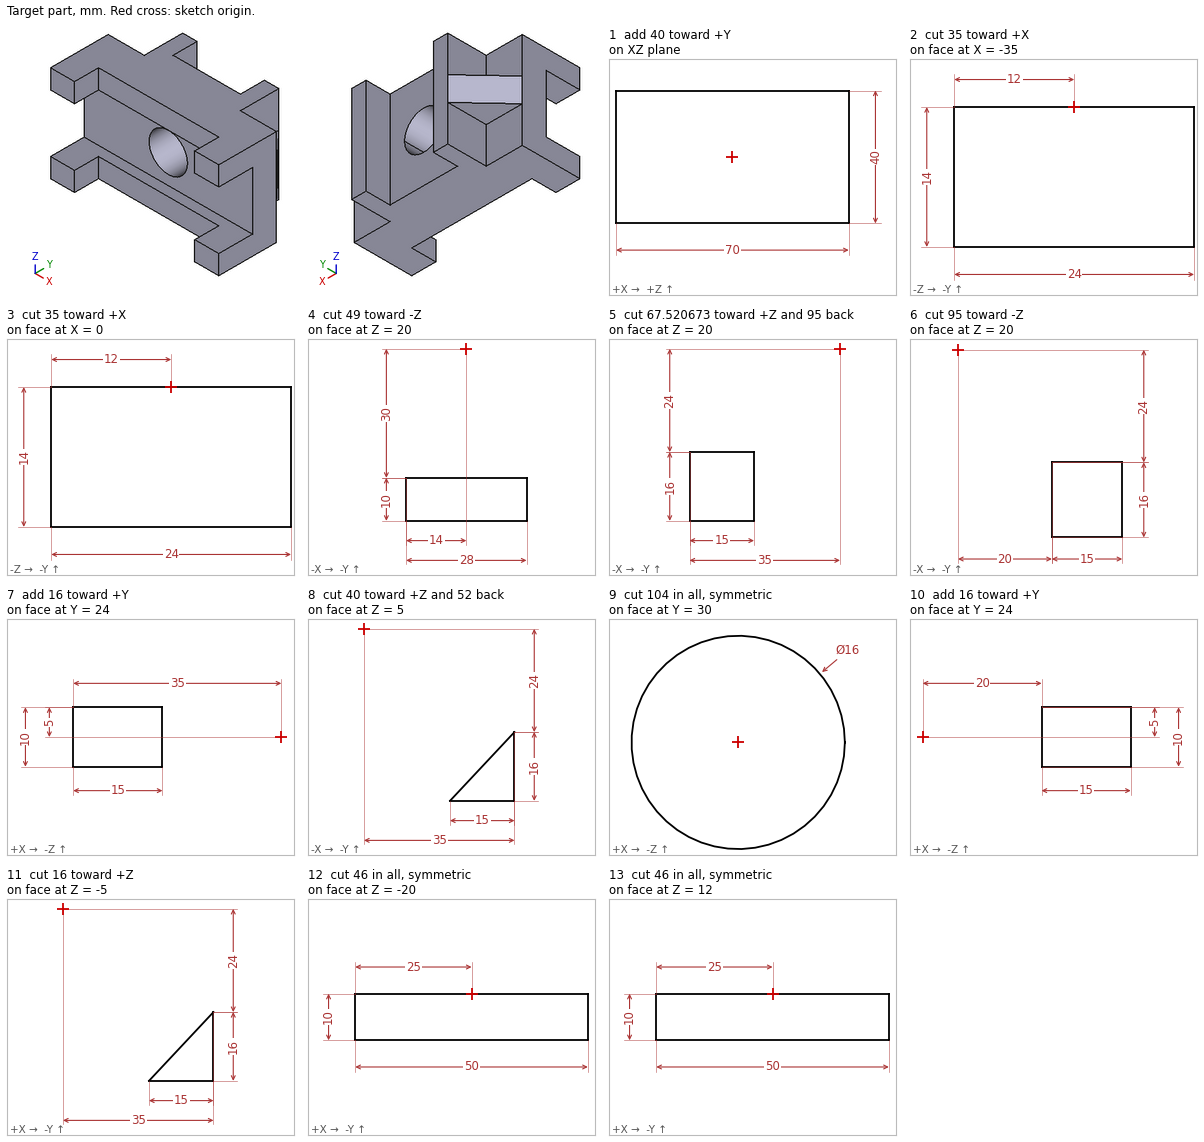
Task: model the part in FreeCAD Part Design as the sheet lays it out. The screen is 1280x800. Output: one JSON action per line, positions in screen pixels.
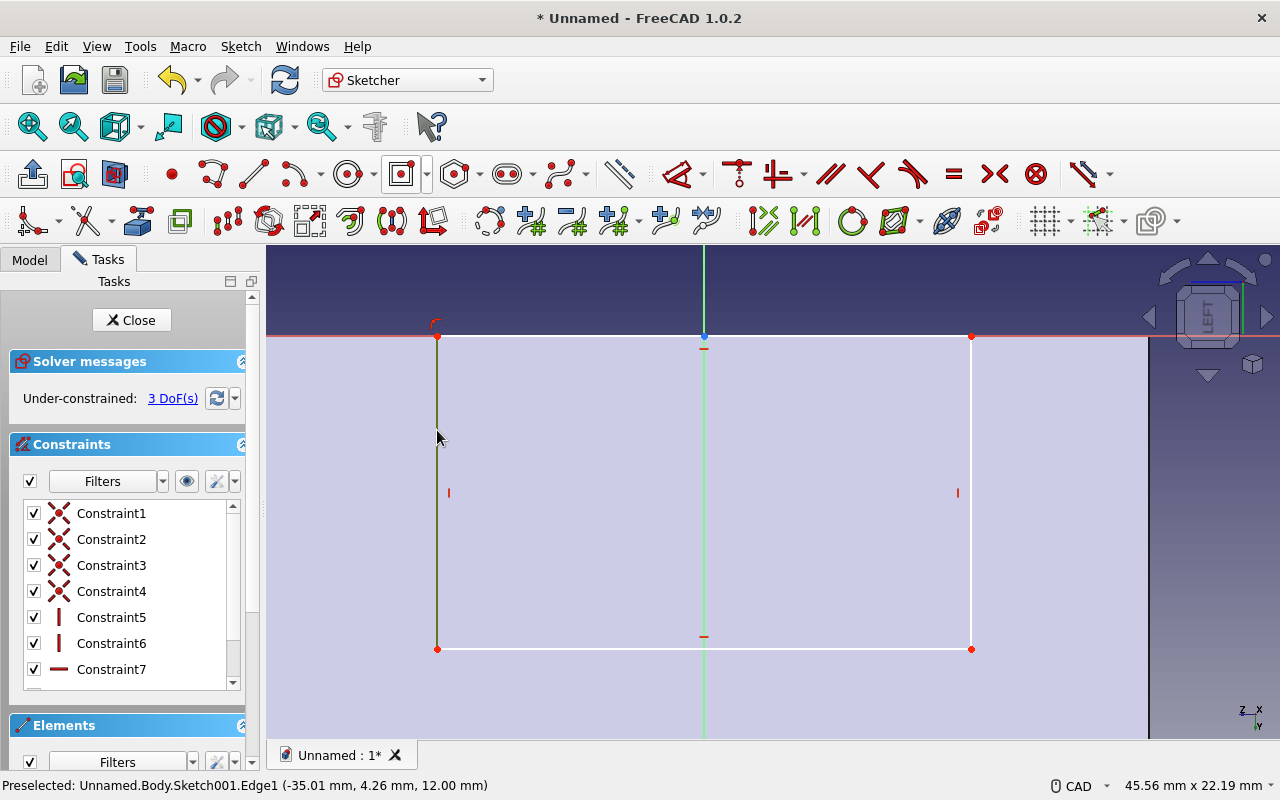
{"action": "key", "text": "i"}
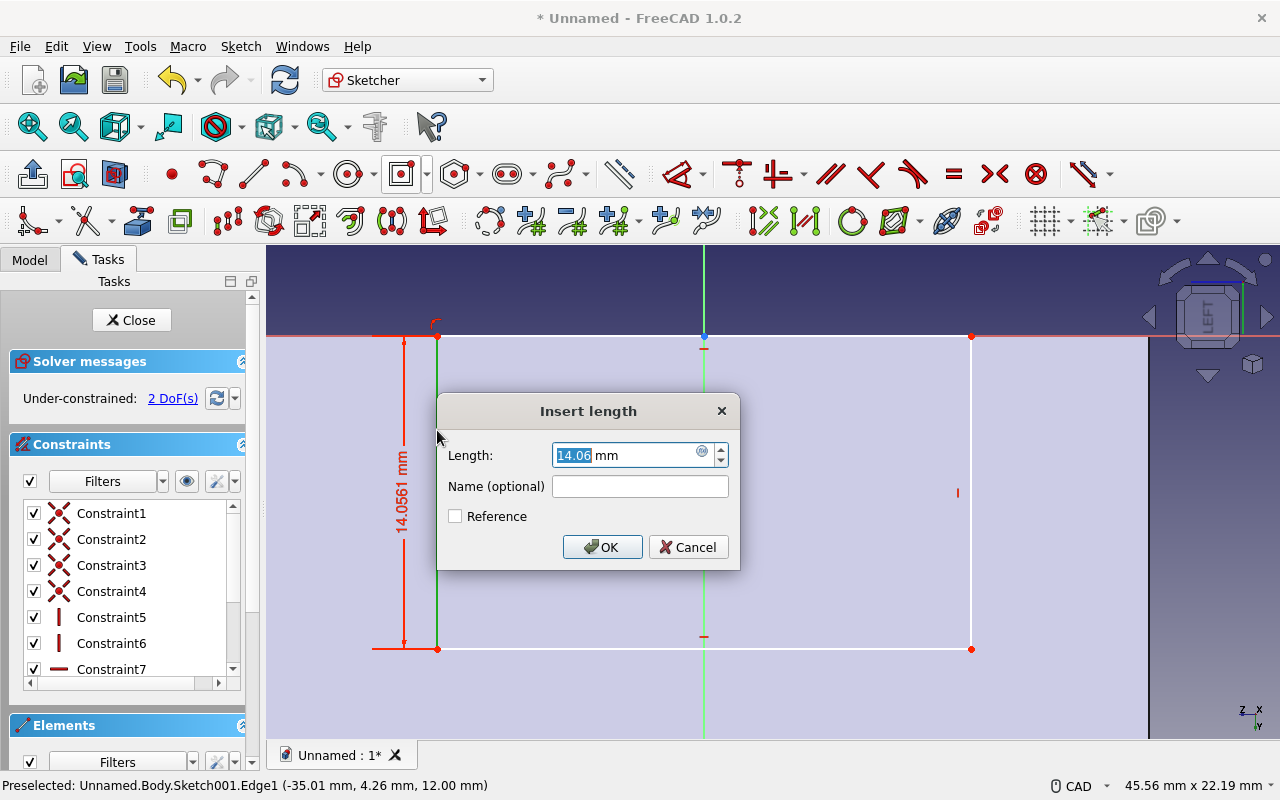
{"action": "type", "text": "14"}
{"action": "key", "text": "Return"}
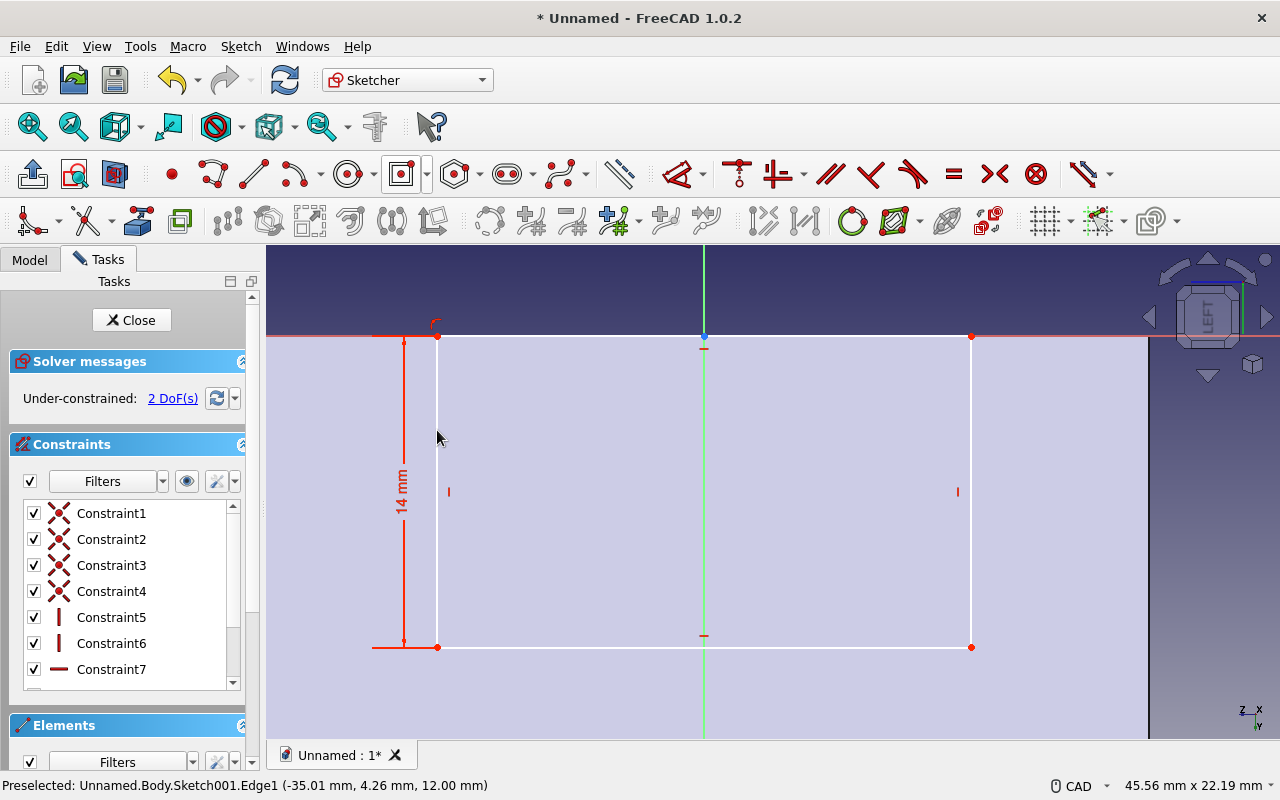
{"action": "left_click", "coordinate": [597, 648]}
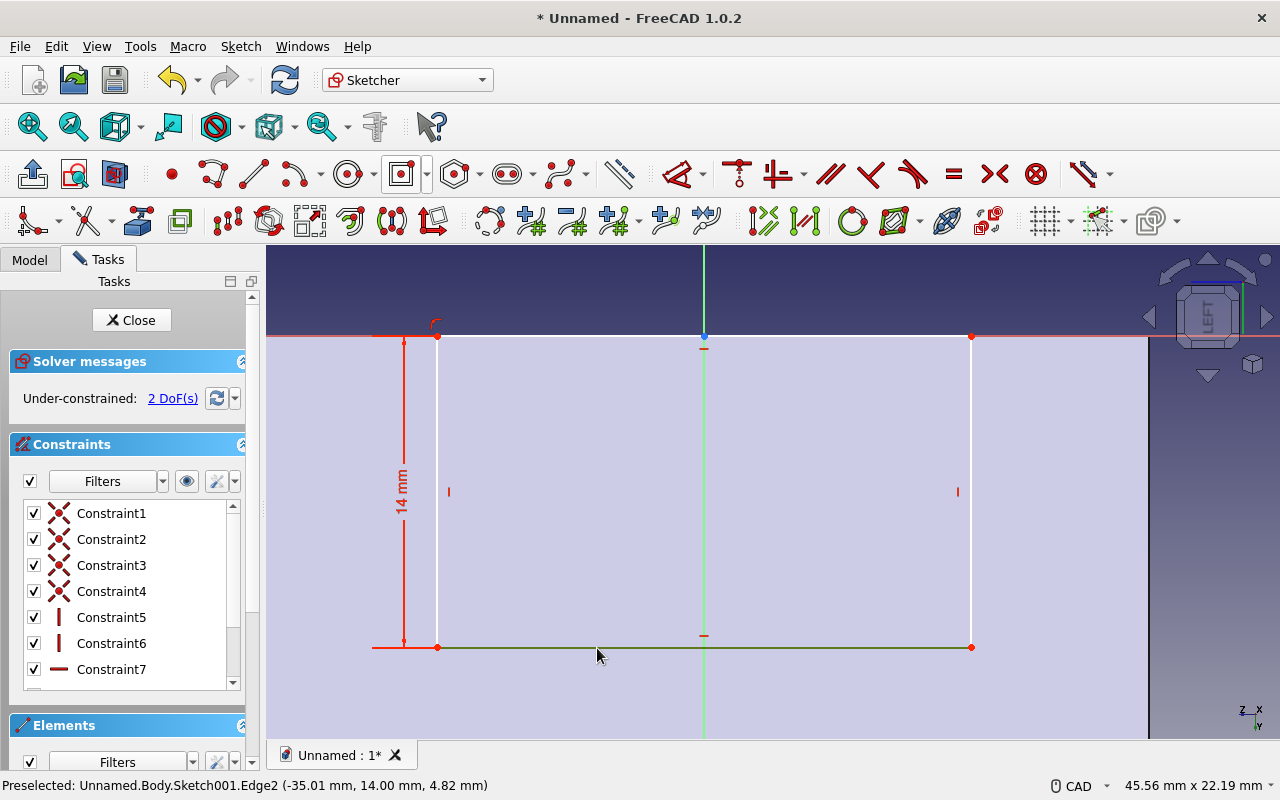
{"action": "key", "text": "l"}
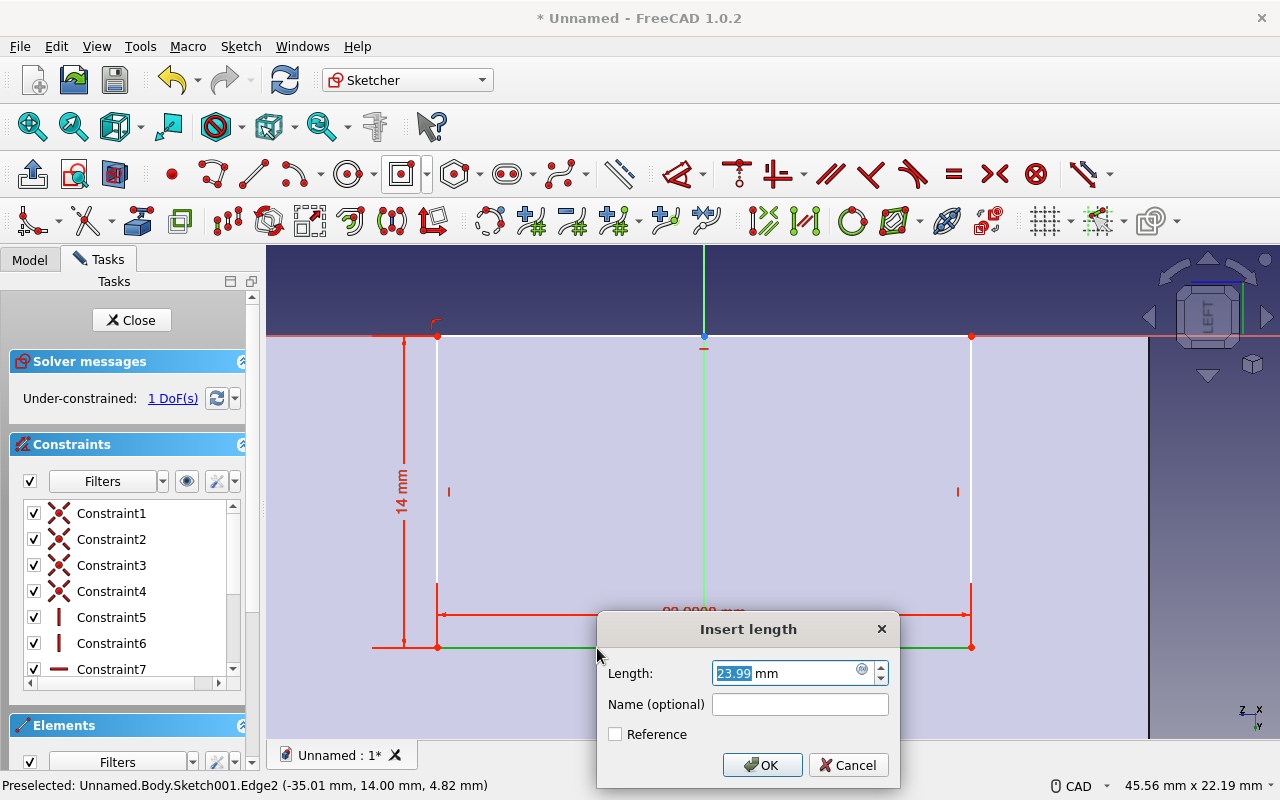
{"action": "type", "text": "24"}
{"action": "key", "text": "Return"}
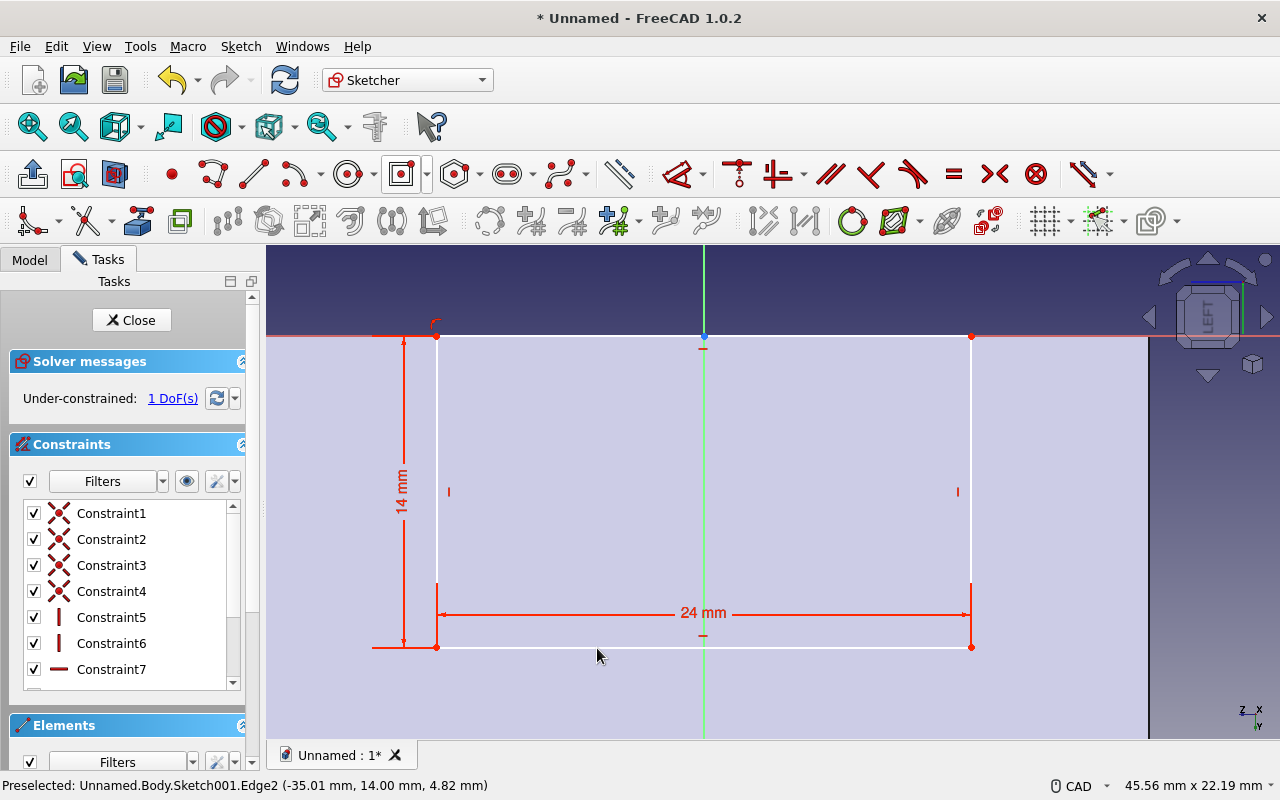
{"action": "left_click", "coordinate": [437, 336]}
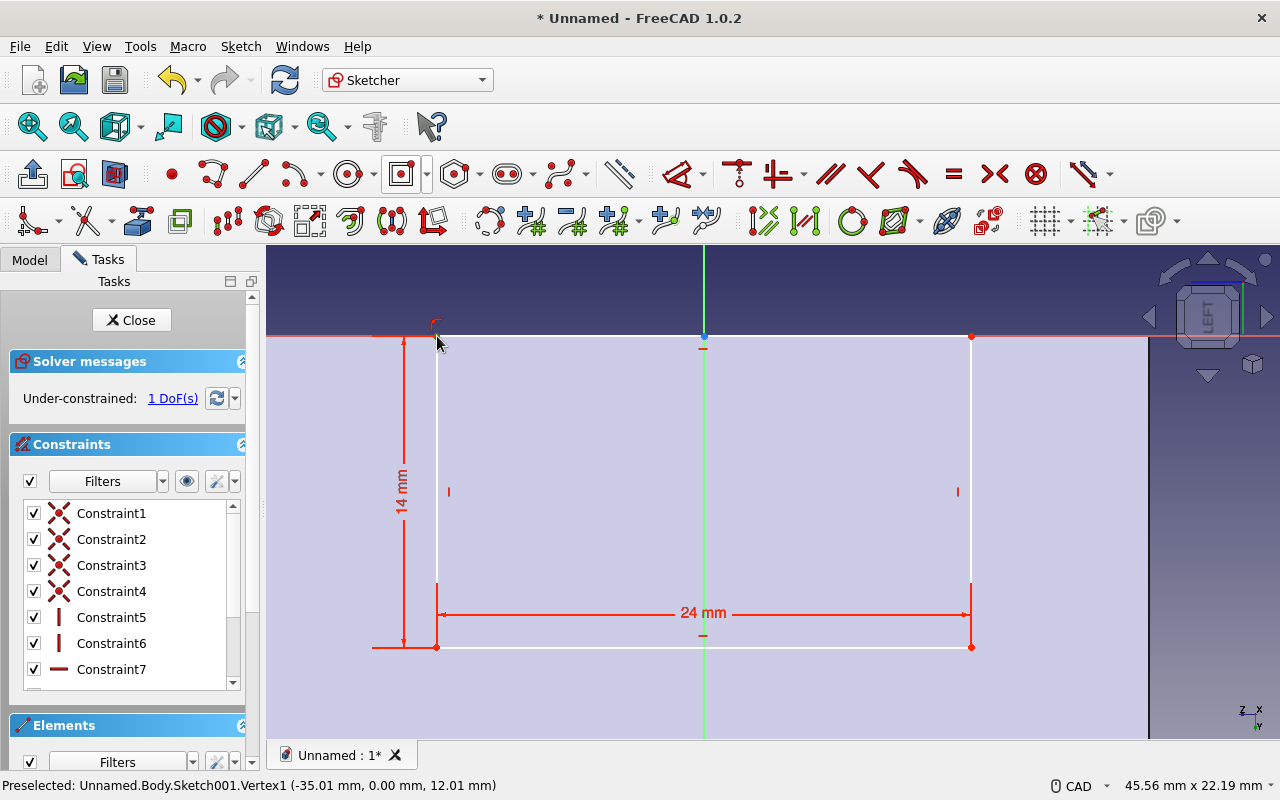
{"action": "key", "text": "l"}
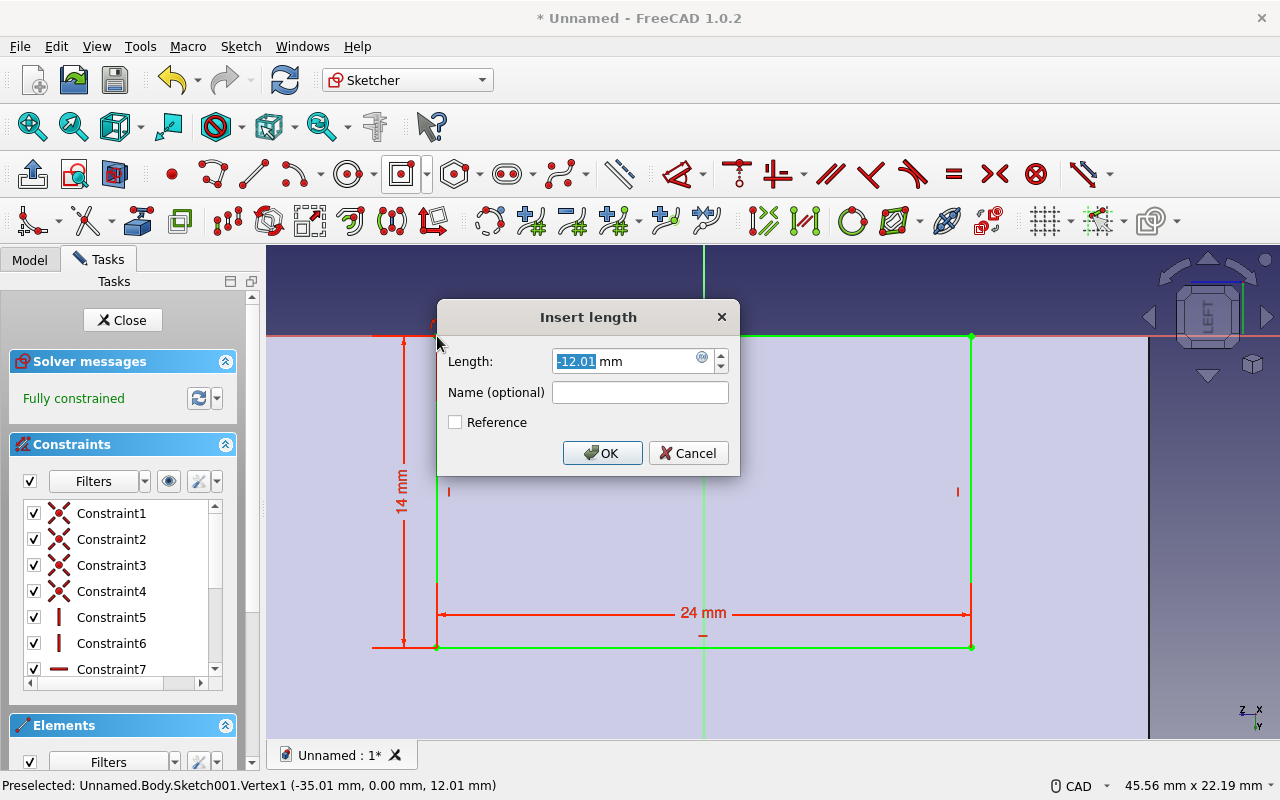
{"action": "type", "text": "-12"}
{"action": "key", "text": "Return"}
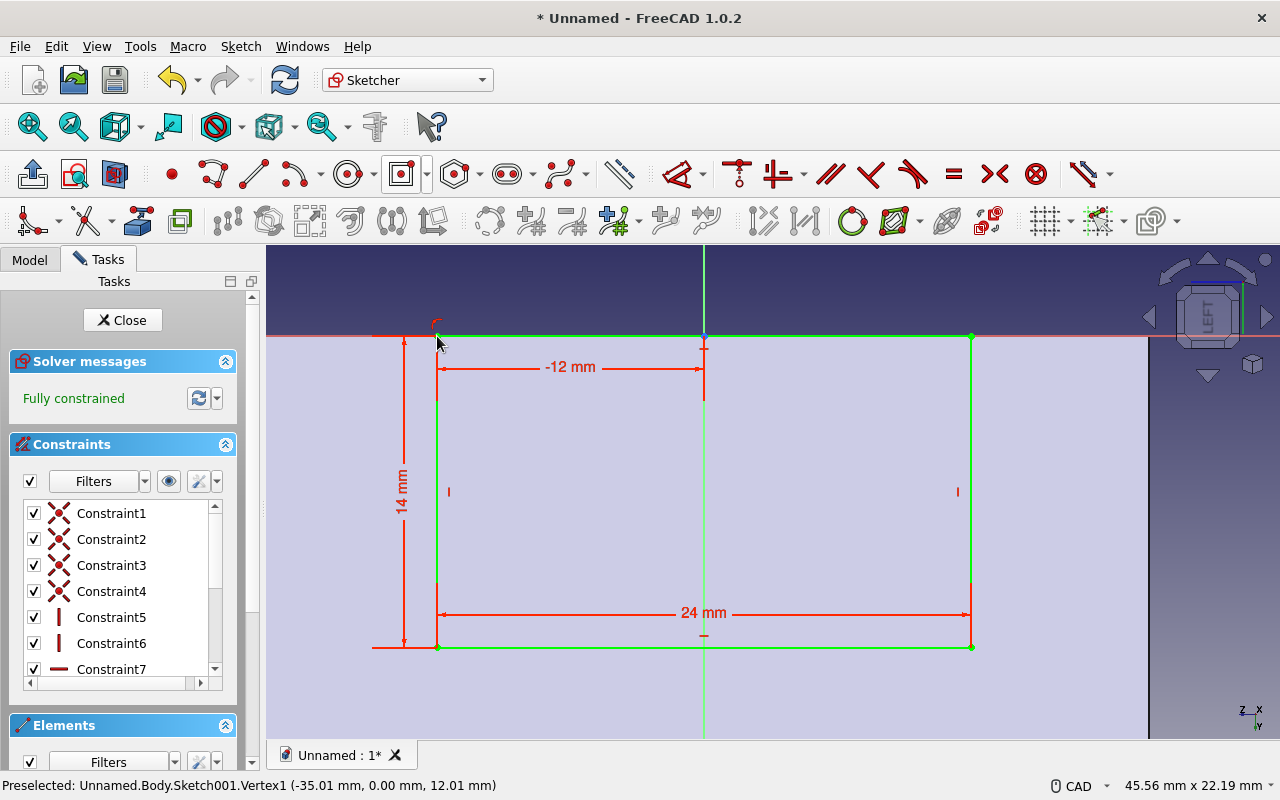
{"action": "left_click", "coordinate": [123, 320]}